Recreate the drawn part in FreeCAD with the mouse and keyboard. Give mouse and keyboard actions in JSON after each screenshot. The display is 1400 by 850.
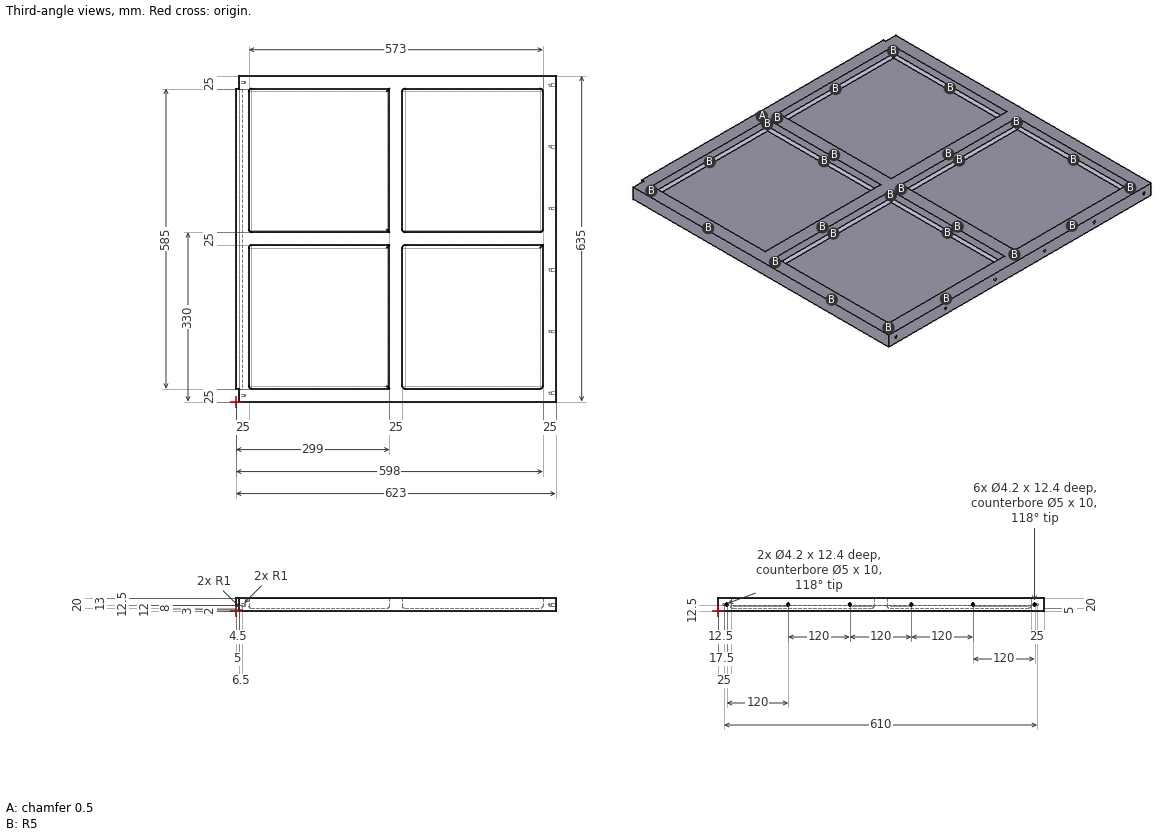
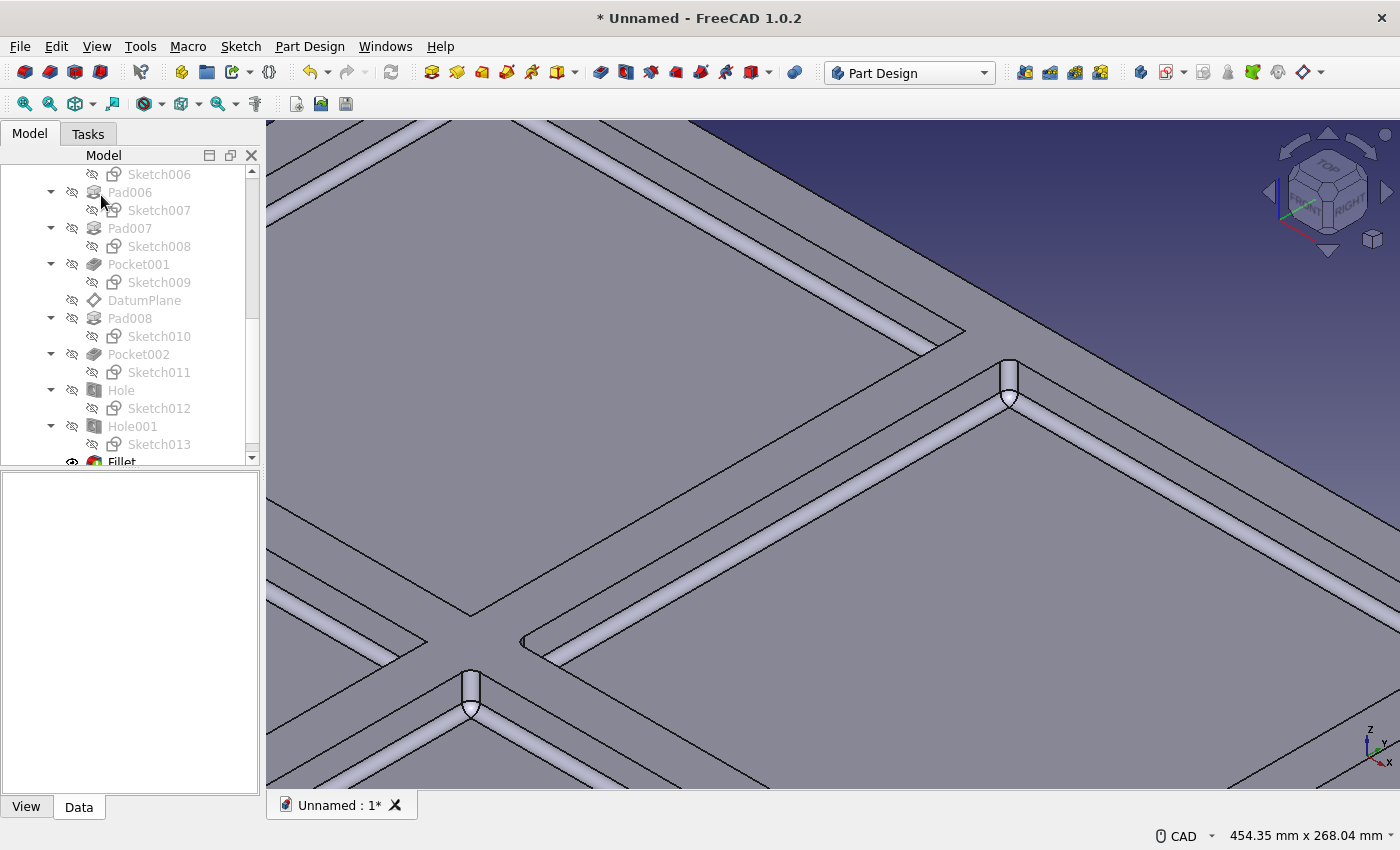
{"action": "left_click", "coordinate": [25, 104]}